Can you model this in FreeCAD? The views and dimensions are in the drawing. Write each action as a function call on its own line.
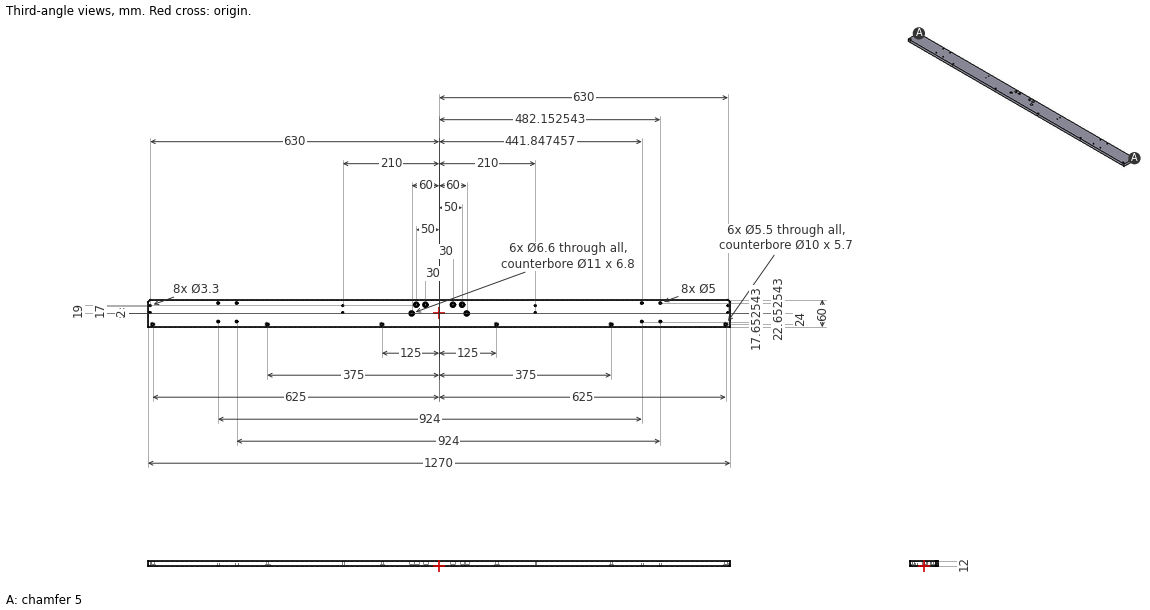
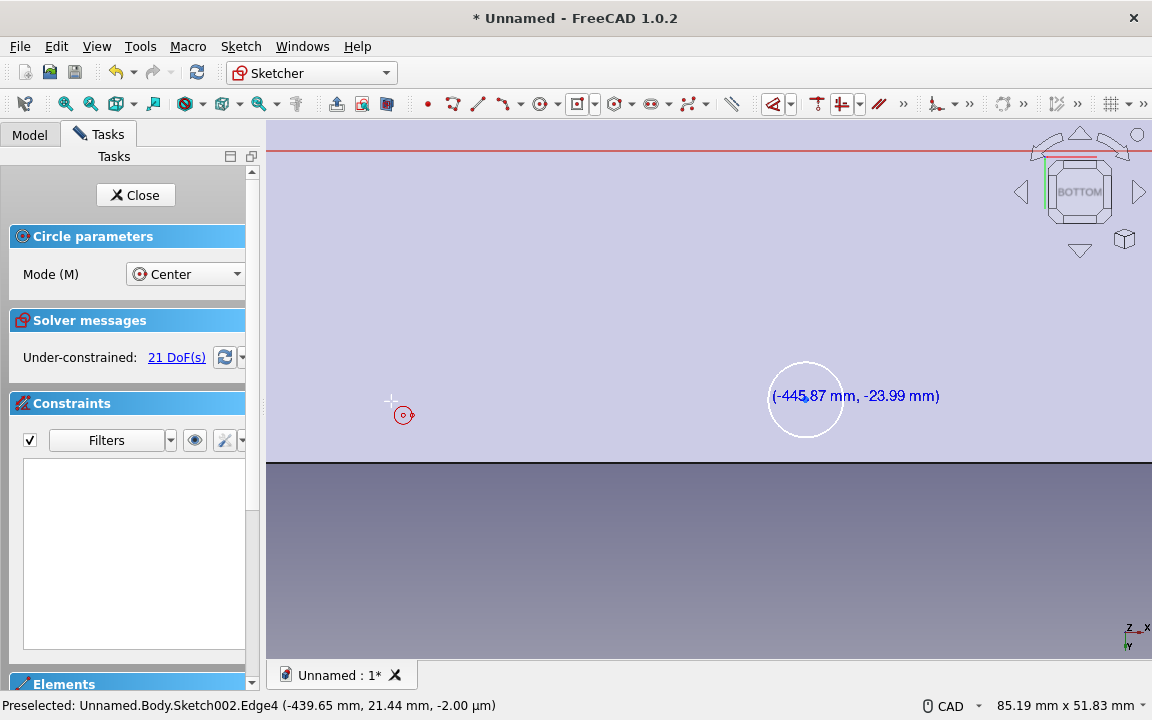
scroll(391, 401, down, 15)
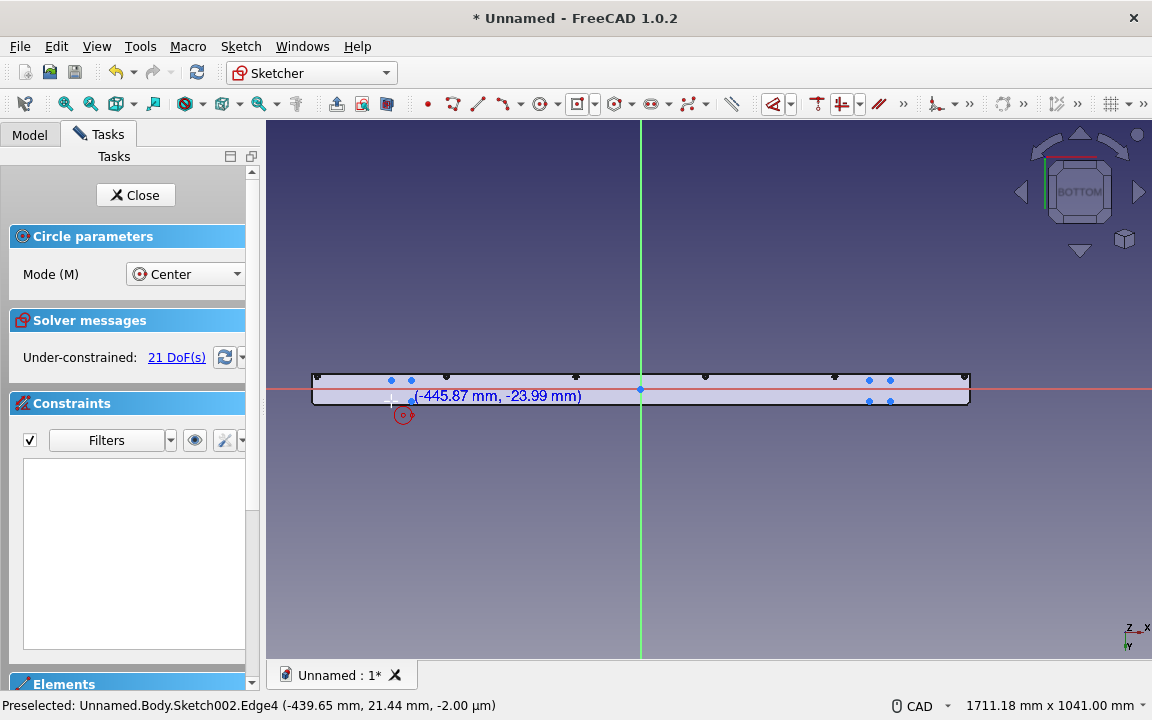
scroll(391, 401, up, 2)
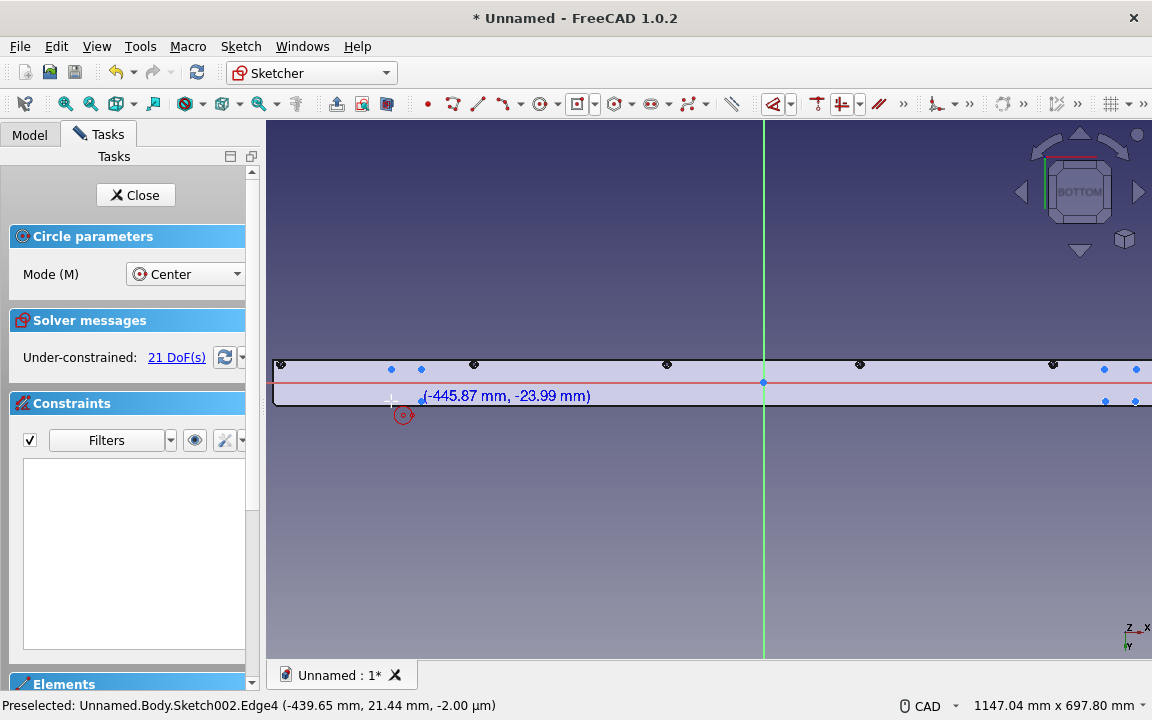
click(391, 400)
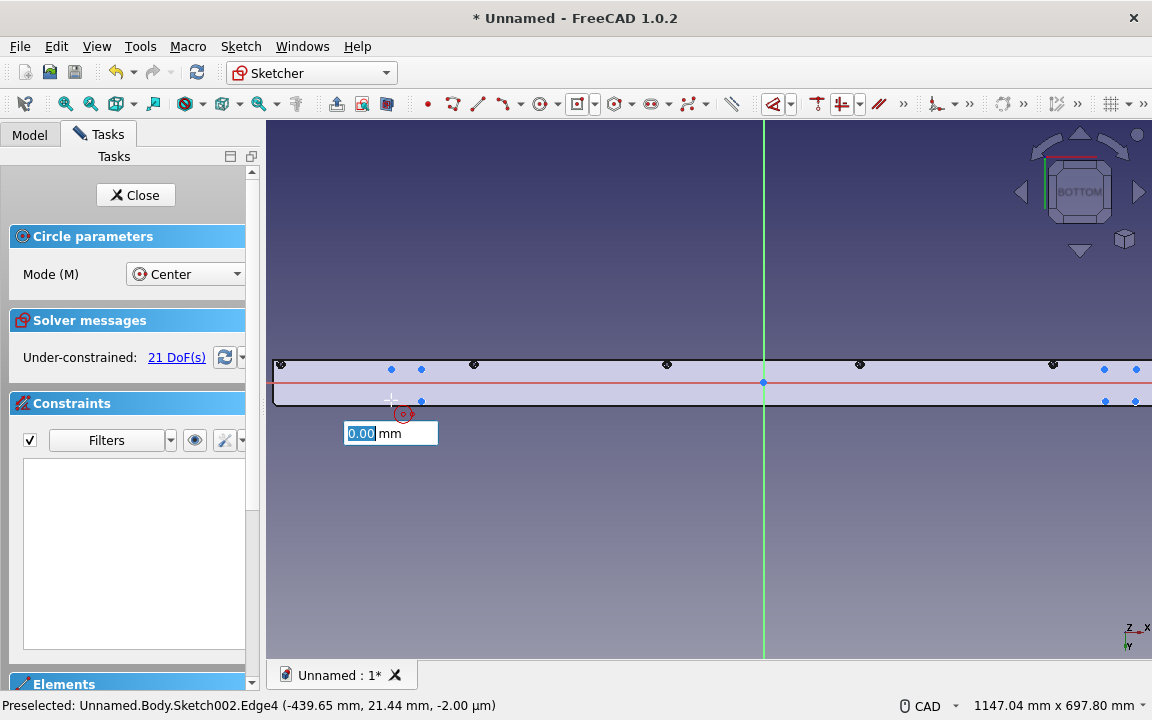
scroll(392, 399, up, 11)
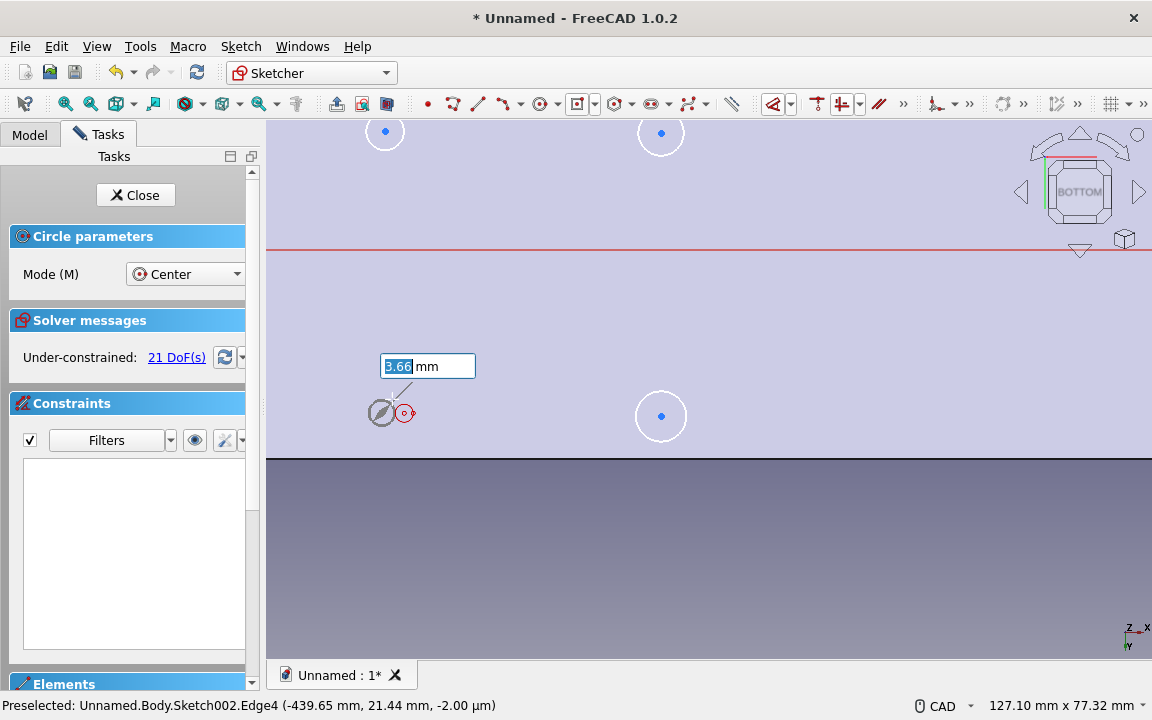
click(395, 395)
key(Escape)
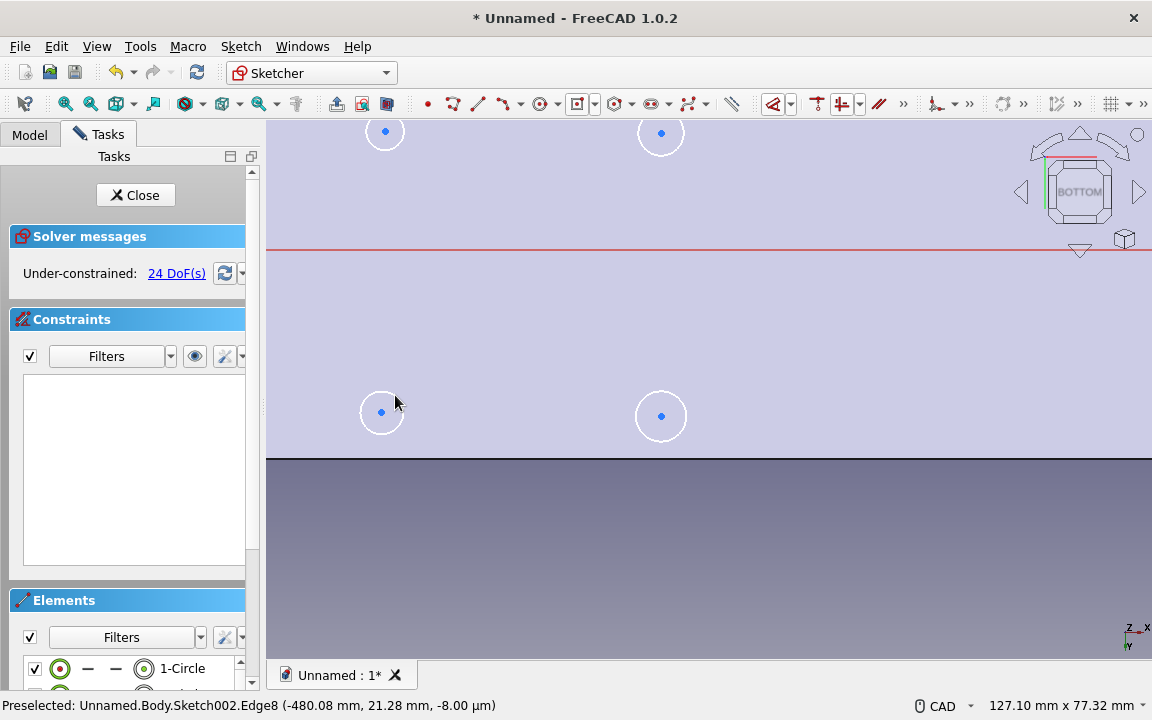
scroll(391, 399, down, 13)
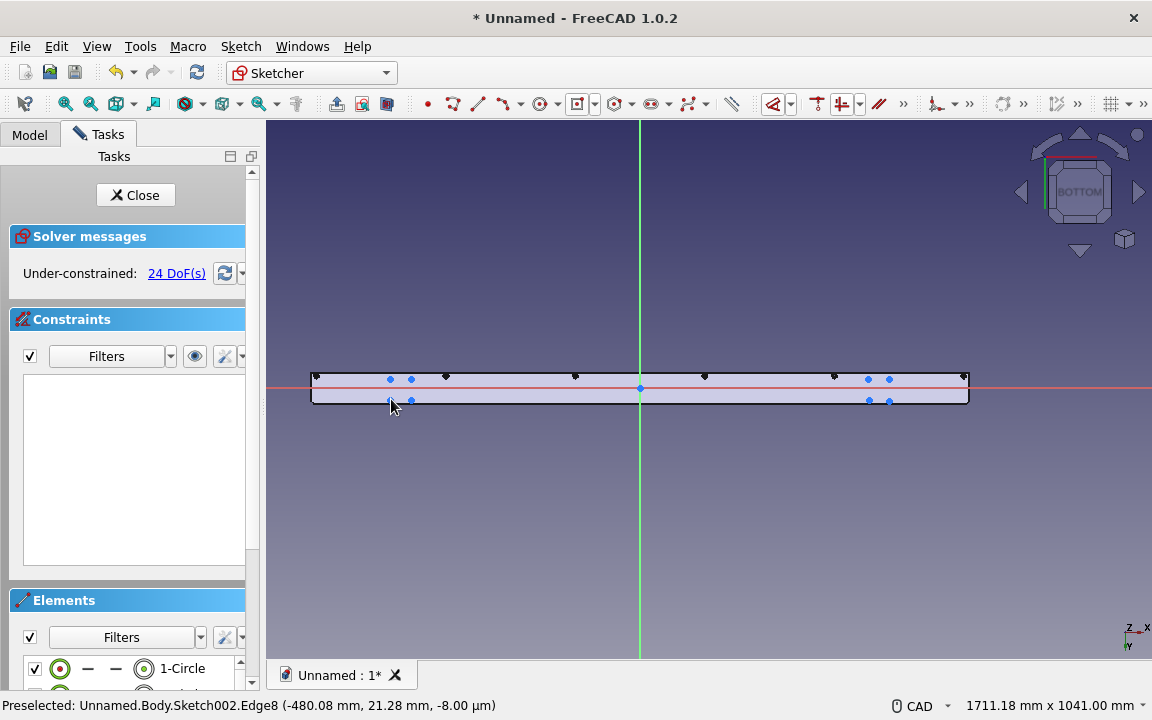
scroll(891, 400, up, 10)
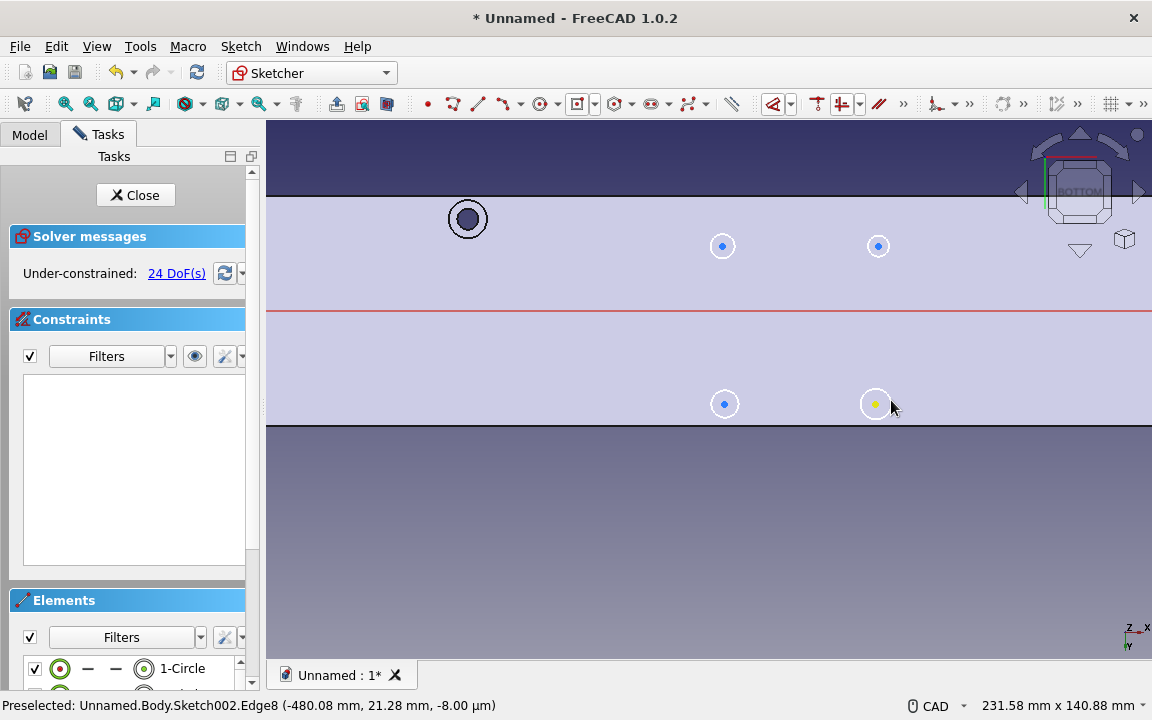
click(887, 393)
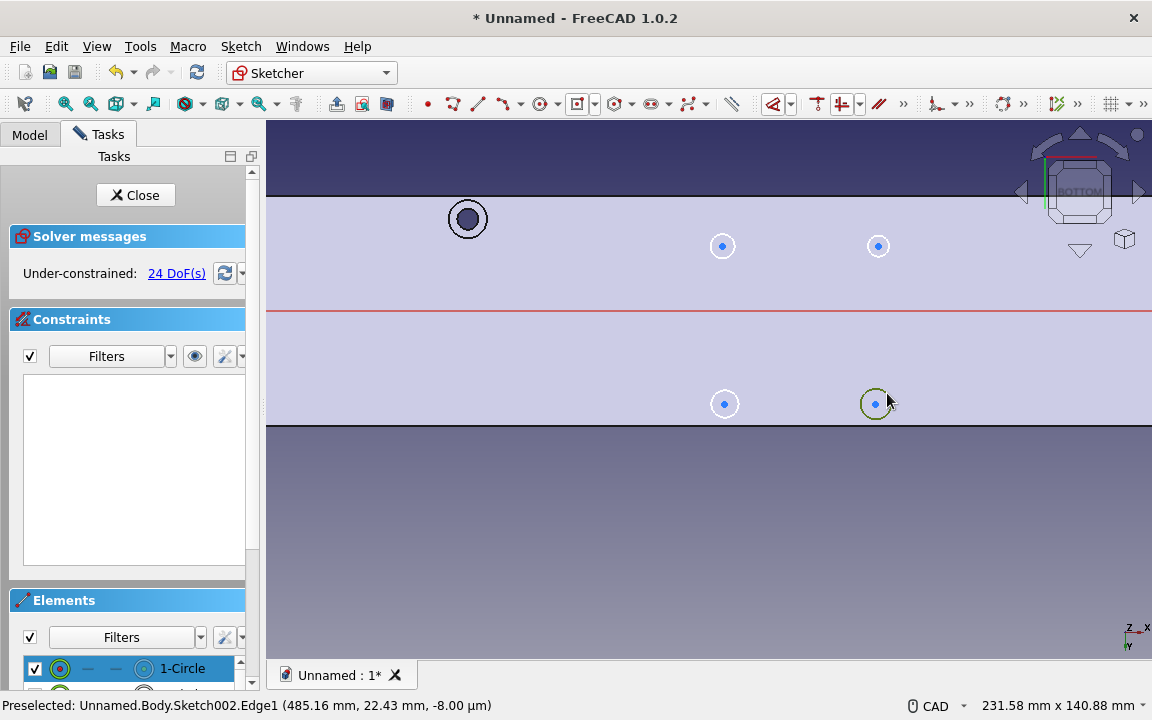
click(735, 394)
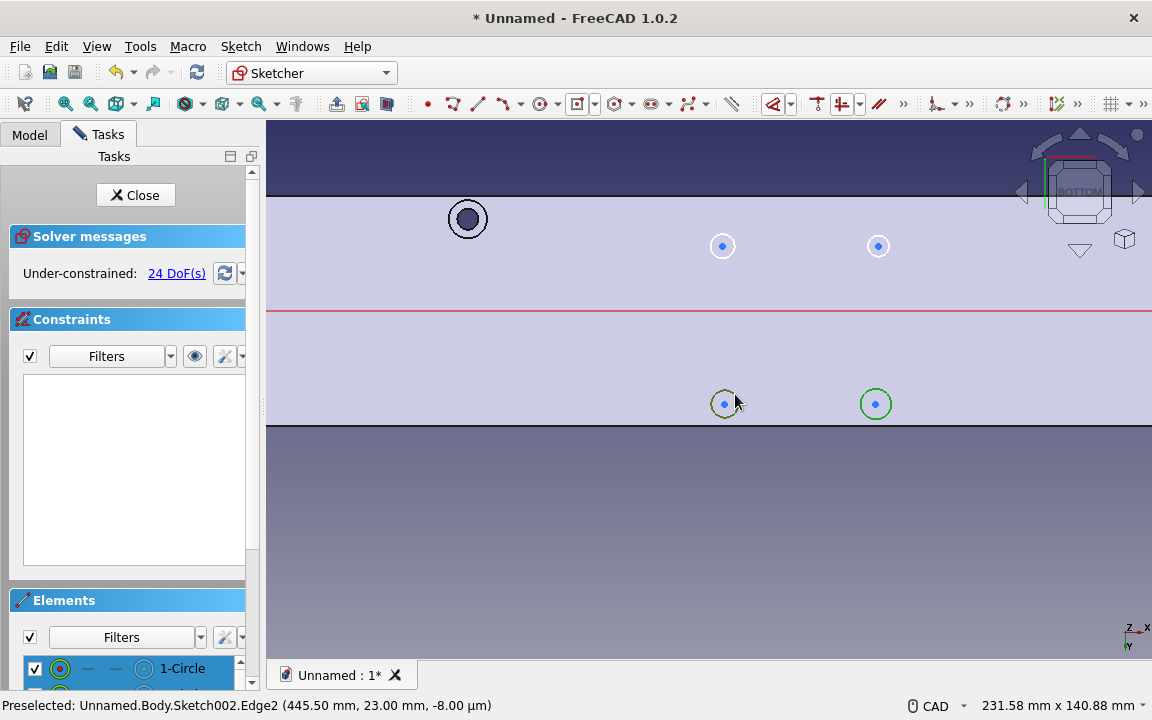
click(731, 238)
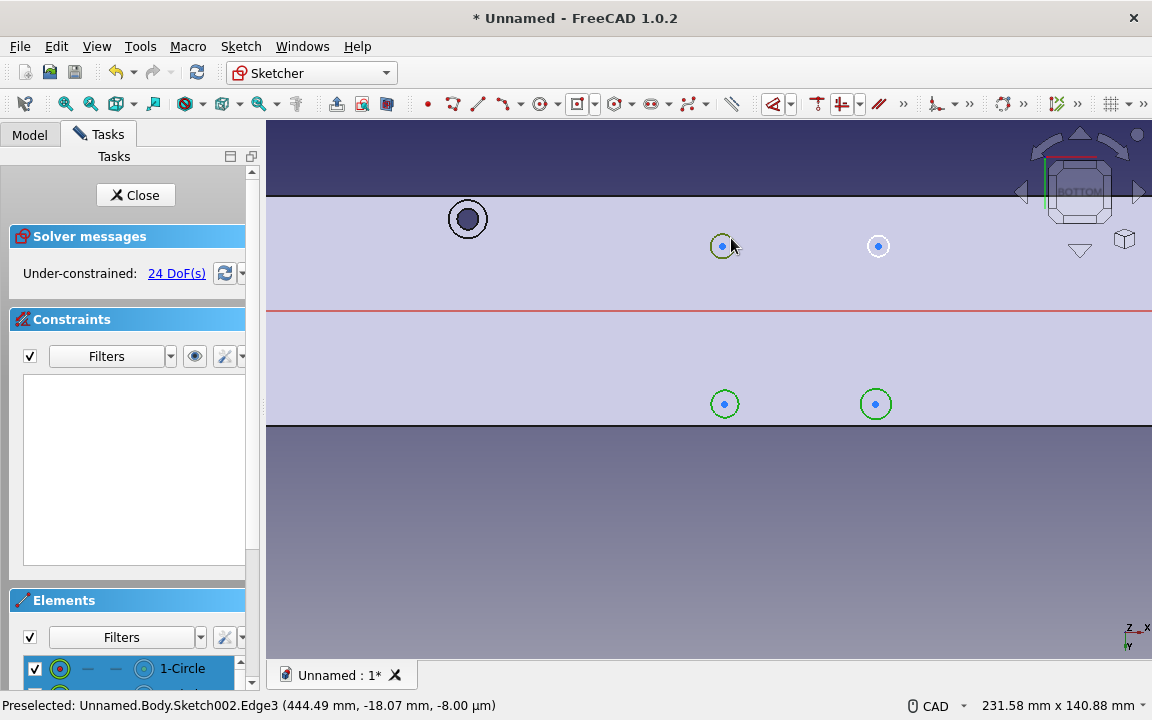
scroll(886, 239, up, 2)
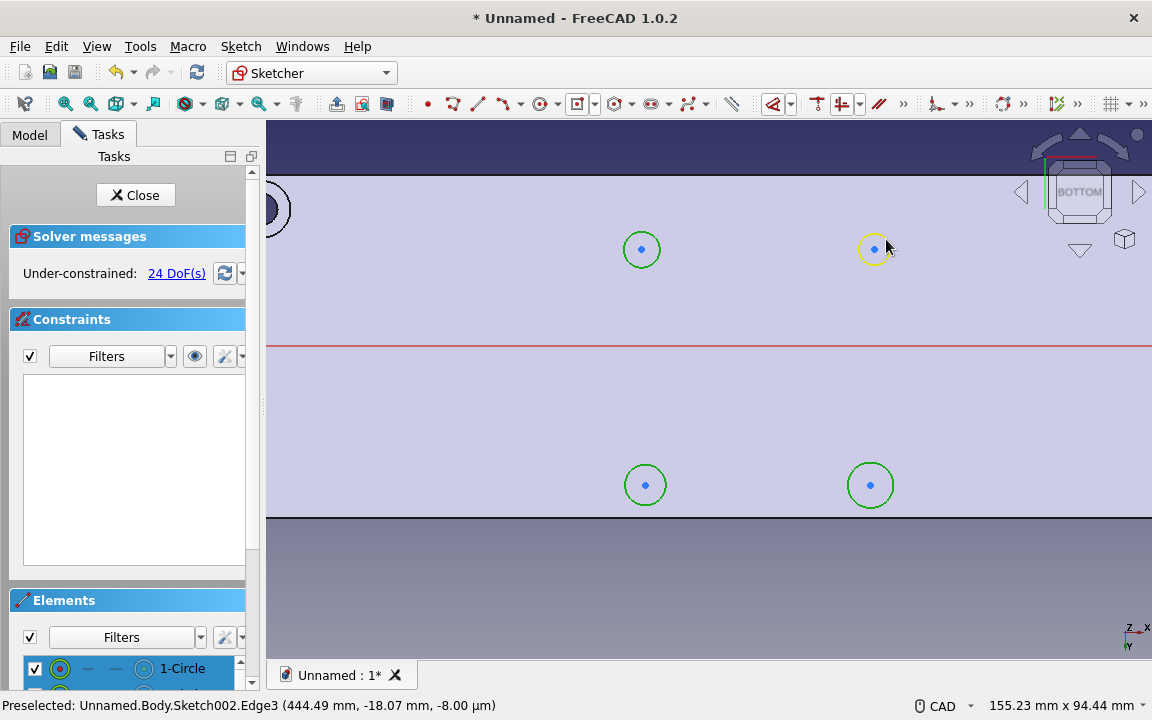
click(886, 238)